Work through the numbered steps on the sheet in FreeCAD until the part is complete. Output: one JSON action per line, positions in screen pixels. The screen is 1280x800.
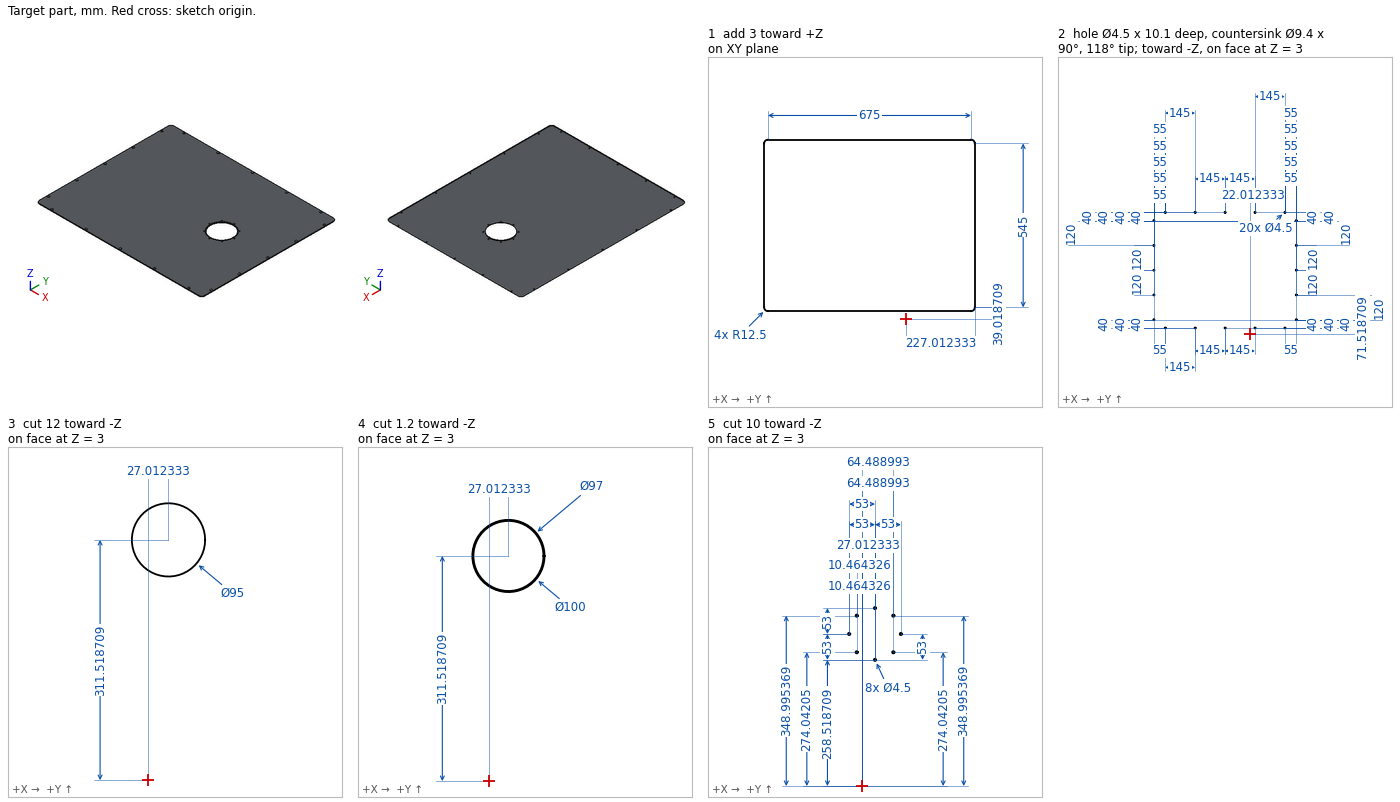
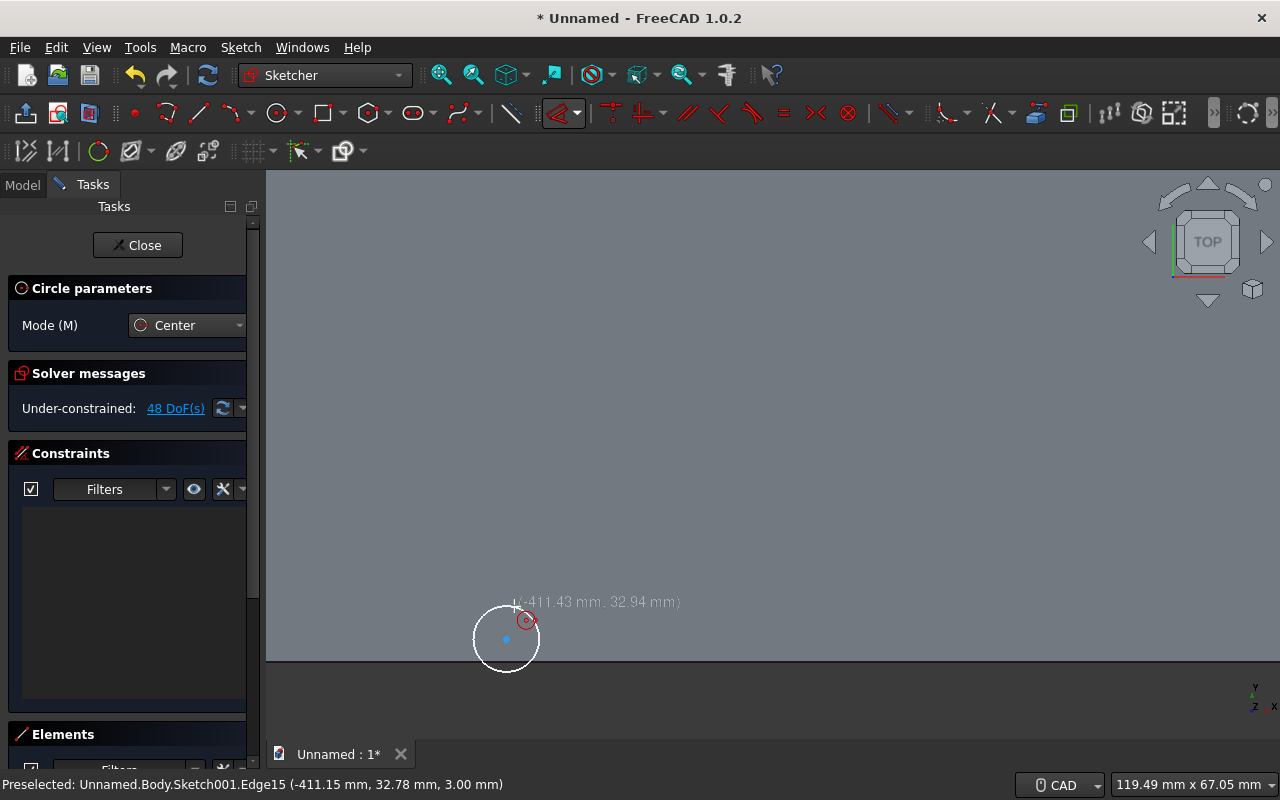
{"action": "scroll", "coordinate": [523, 622], "scroll_direction": "down", "scroll_amount": 13}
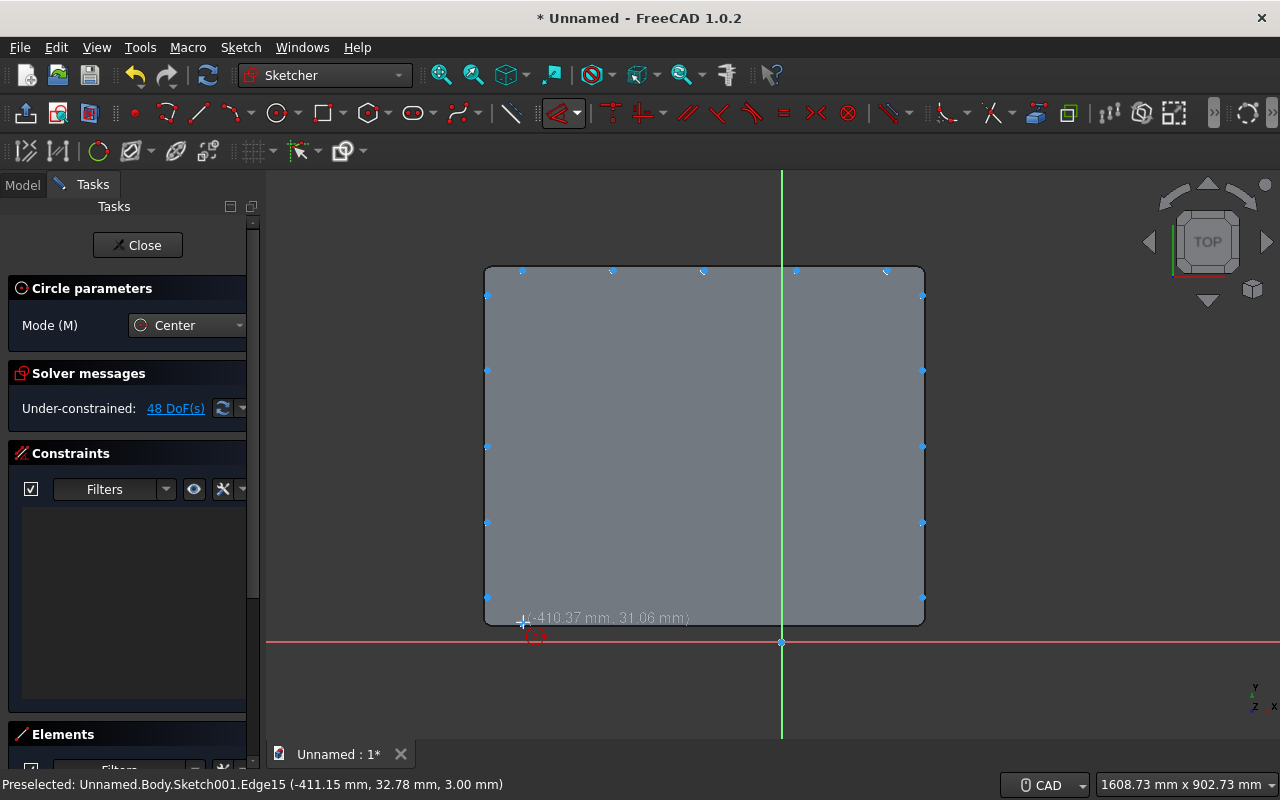
{"action": "scroll", "coordinate": [613, 623], "scroll_direction": "up", "scroll_amount": 14}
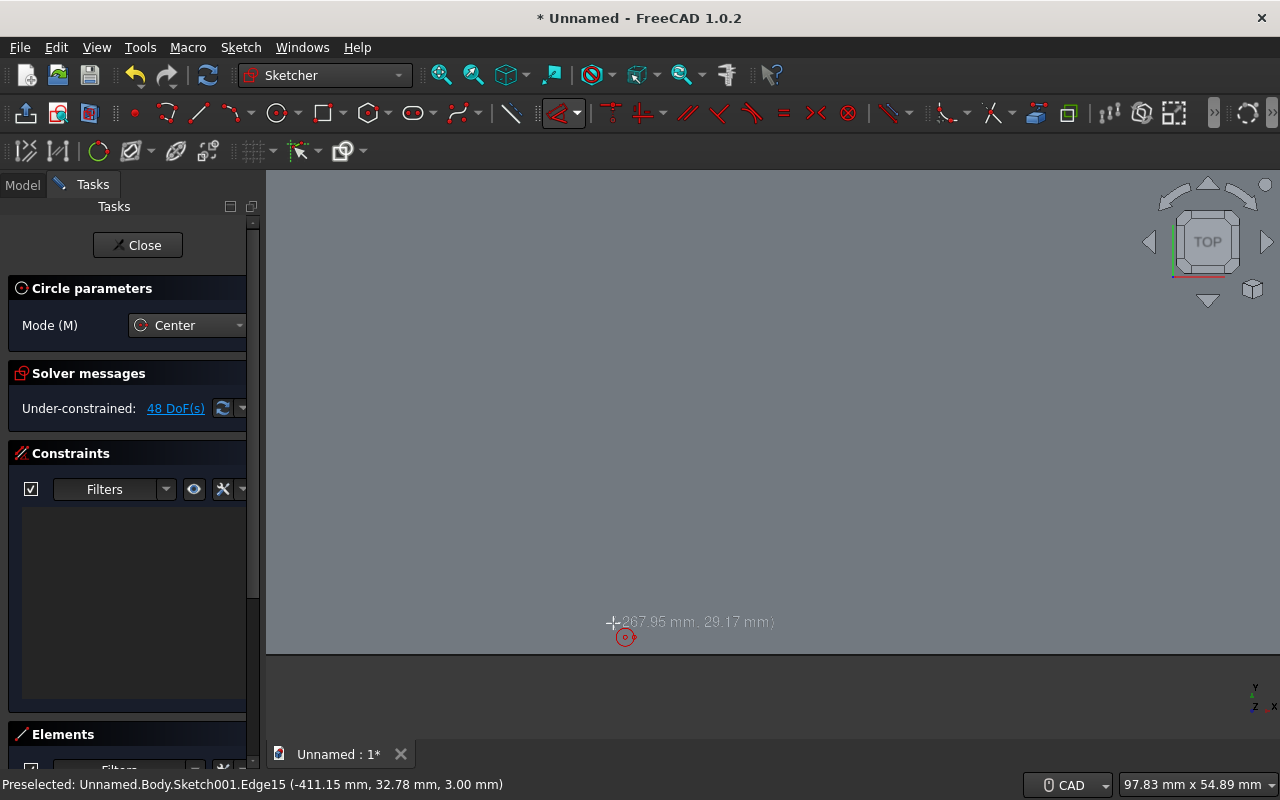
{"action": "scroll", "coordinate": [613, 623], "scroll_direction": "down", "scroll_amount": 14}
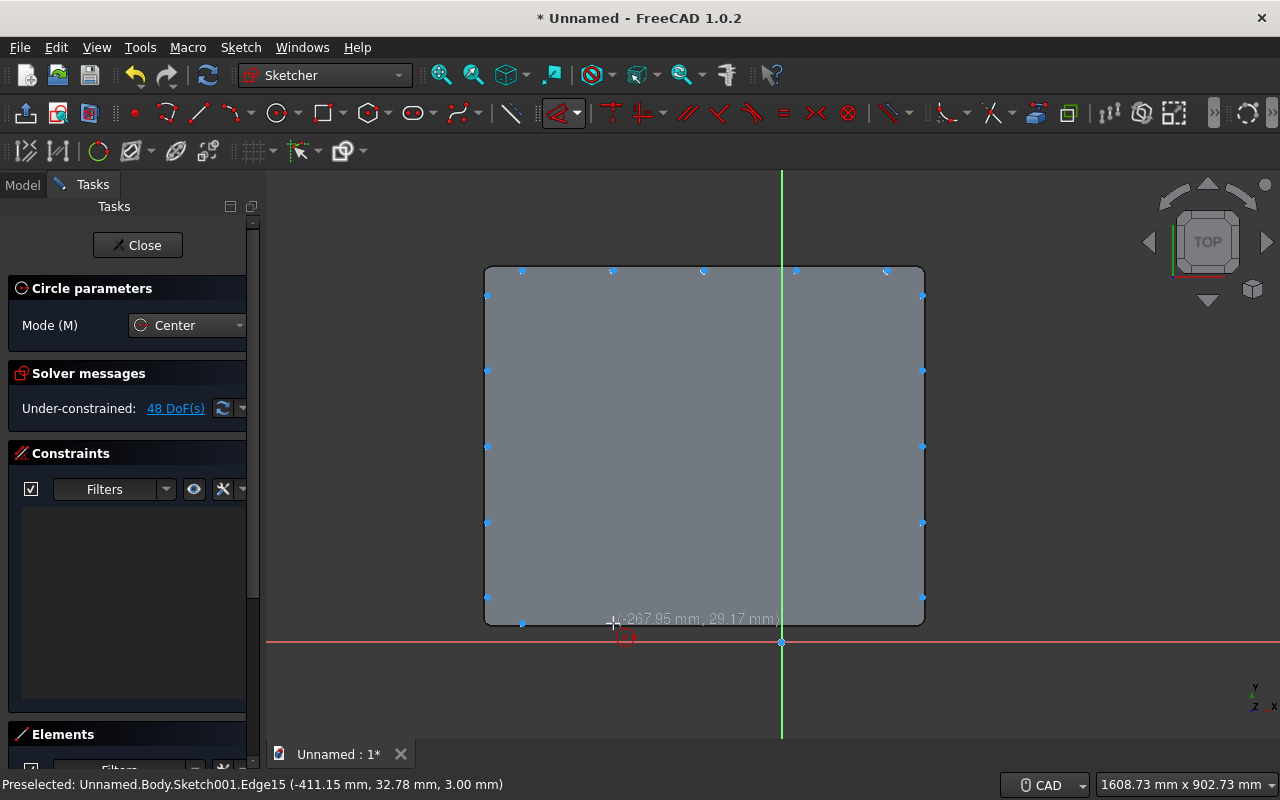
{"action": "left_click", "coordinate": [613, 623]}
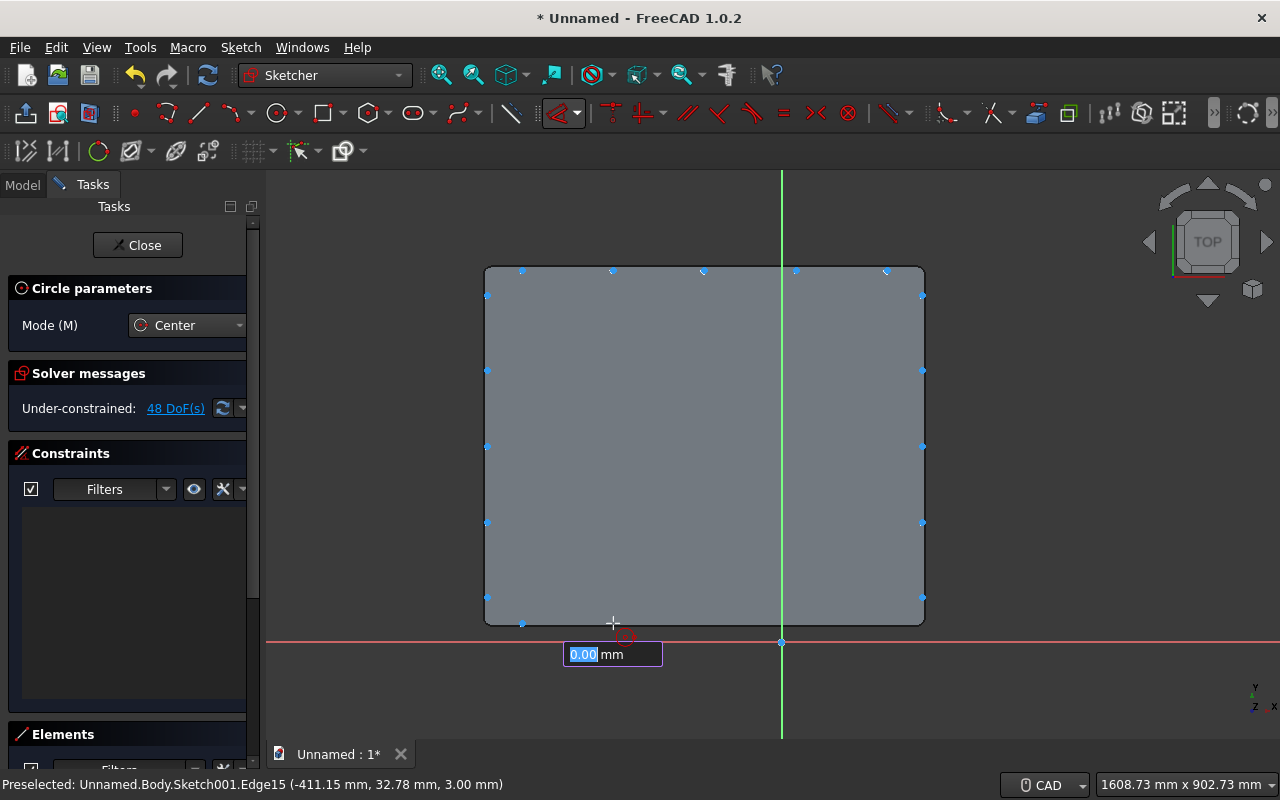
{"action": "scroll", "coordinate": [614, 622], "scroll_direction": "up", "scroll_amount": 13}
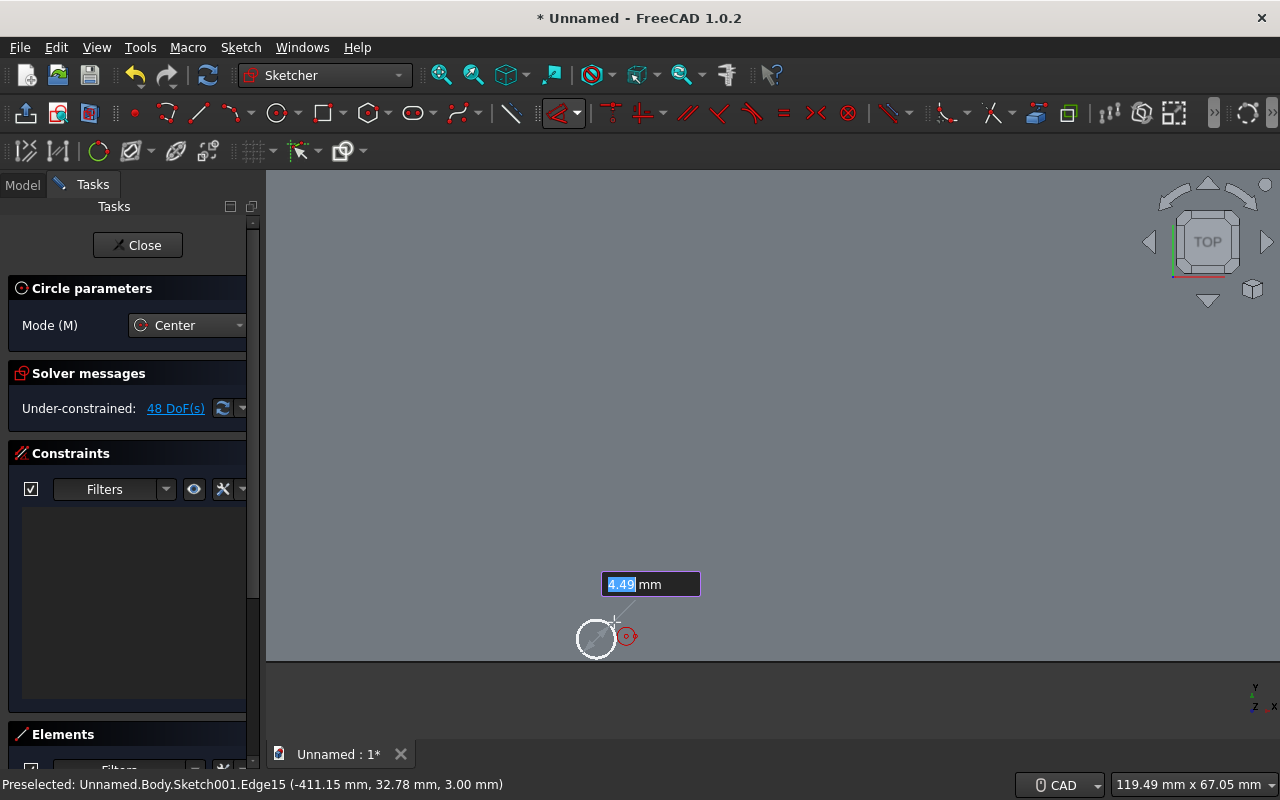
{"action": "left_click", "coordinate": [609, 606]}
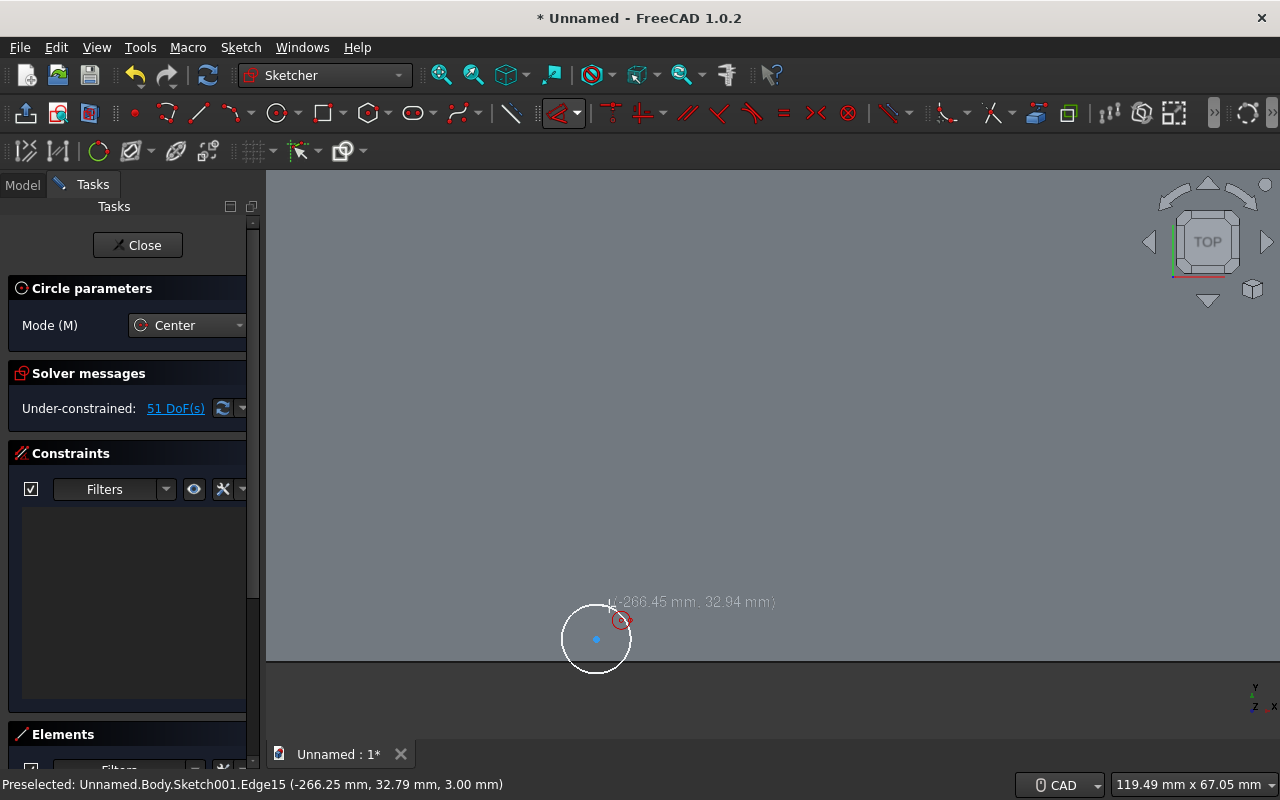
{"action": "scroll", "coordinate": [614, 622], "scroll_direction": "down", "scroll_amount": 13}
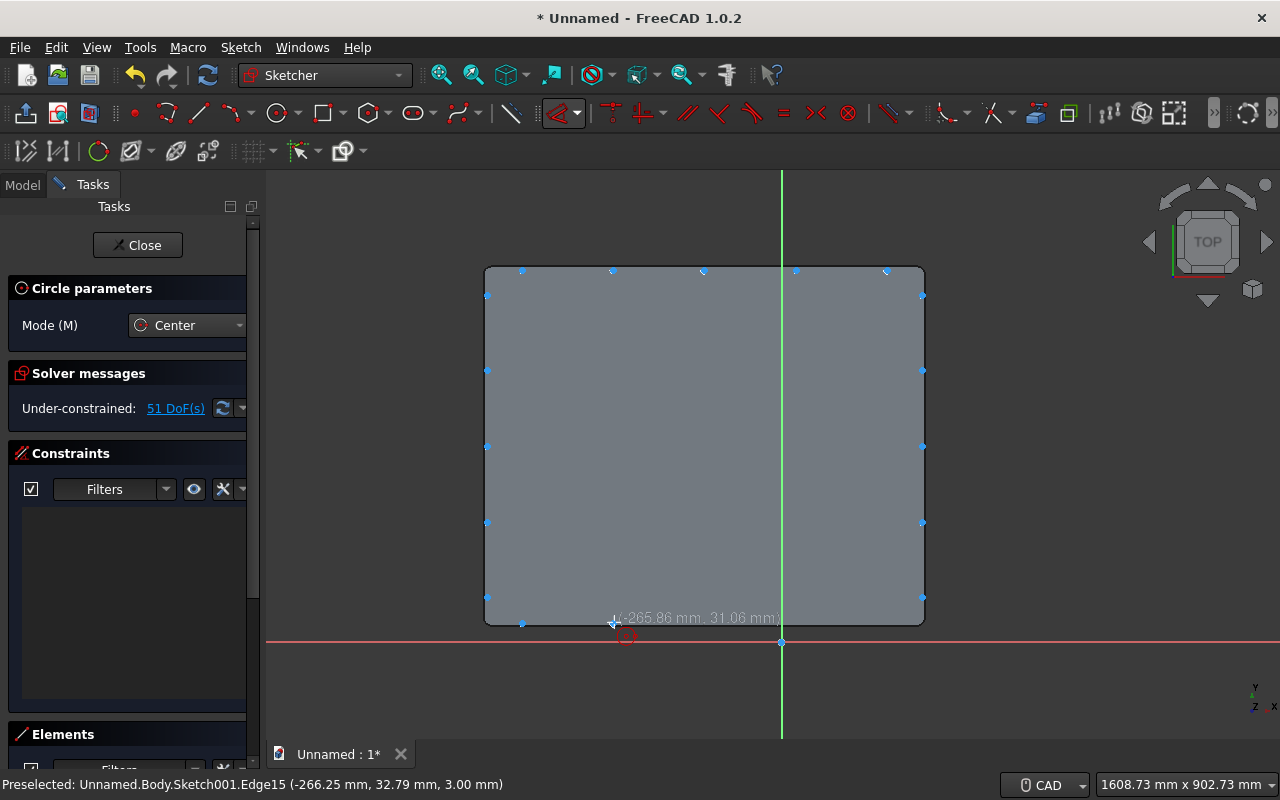
{"action": "scroll", "coordinate": [704, 623], "scroll_direction": "up", "scroll_amount": 14}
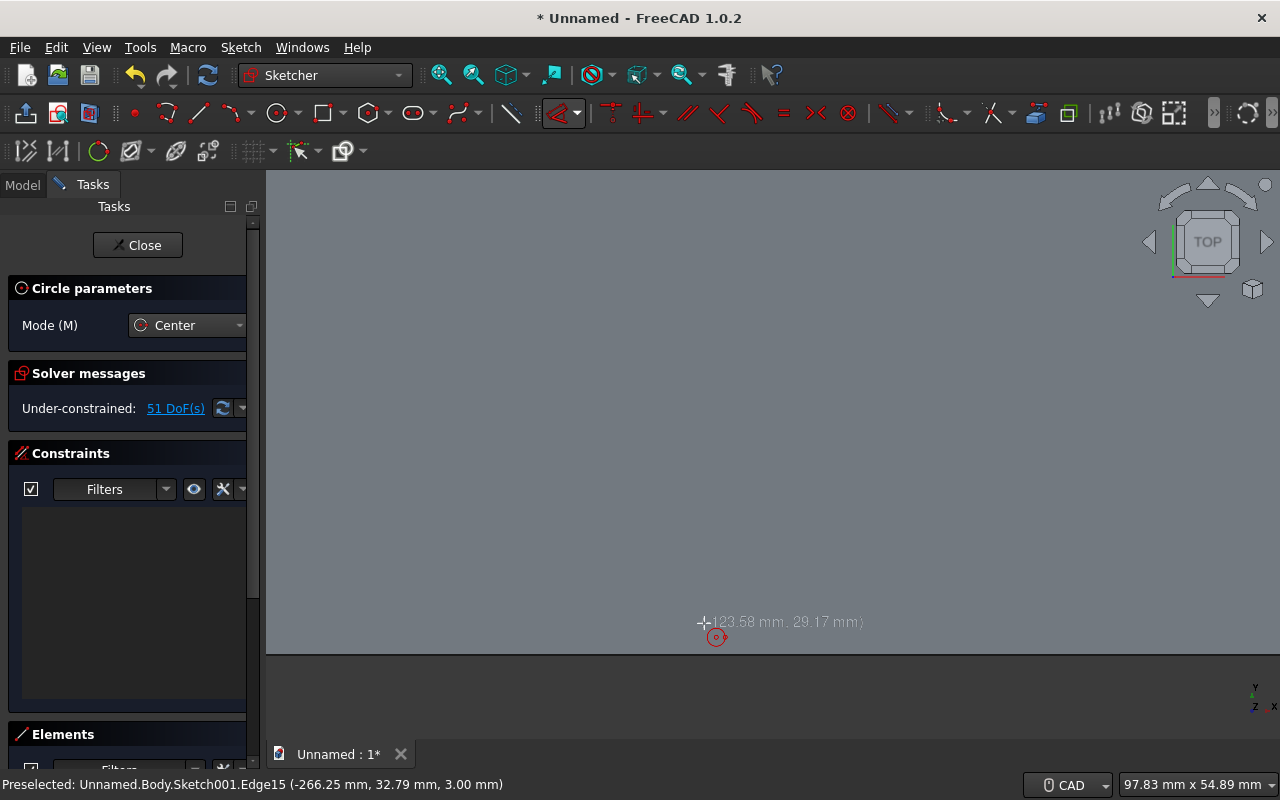
{"action": "scroll", "coordinate": [705, 623], "scroll_direction": "down", "scroll_amount": 14}